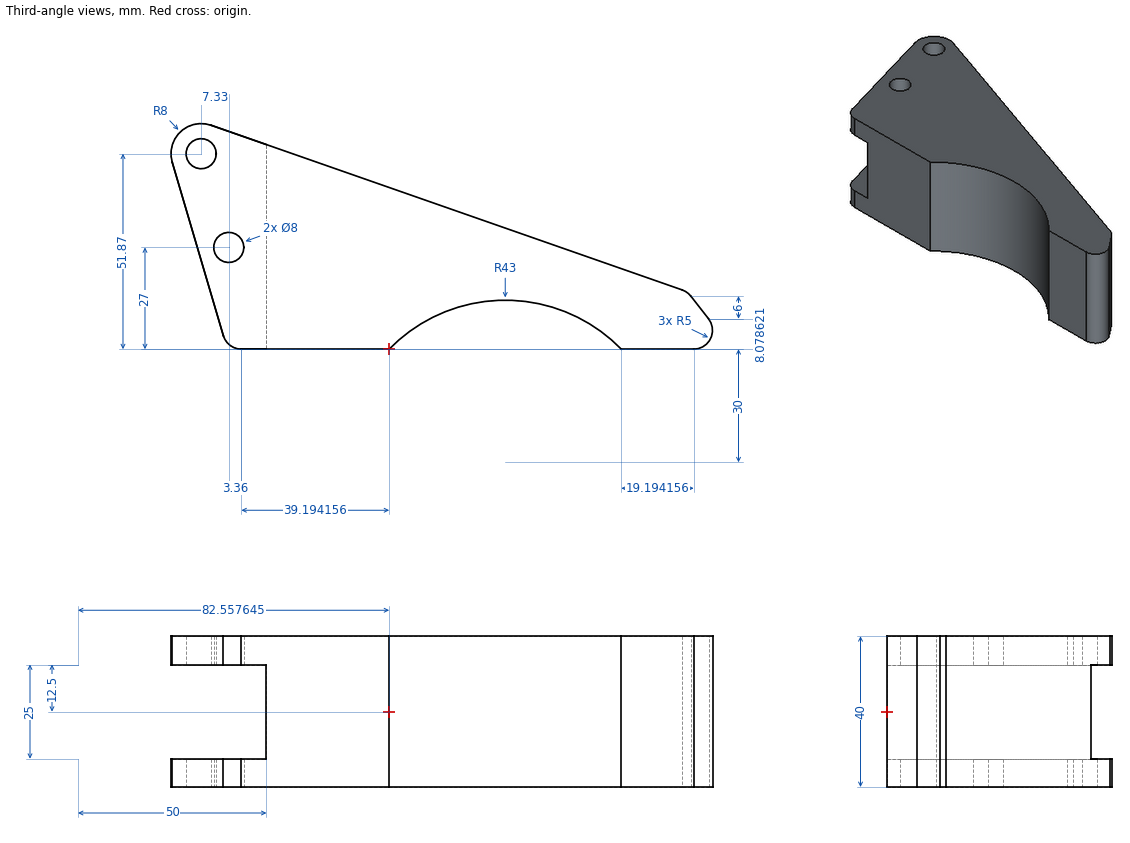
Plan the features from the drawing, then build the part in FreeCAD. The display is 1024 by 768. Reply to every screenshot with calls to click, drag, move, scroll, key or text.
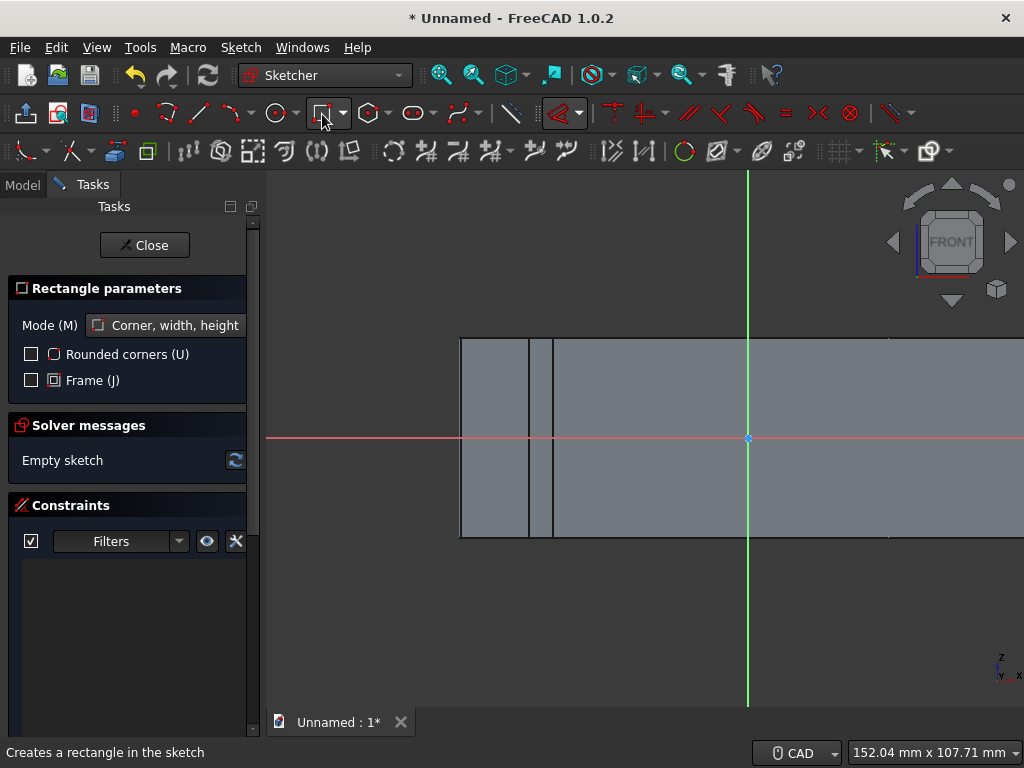
click(336, 376)
click(586, 500)
key(Escape)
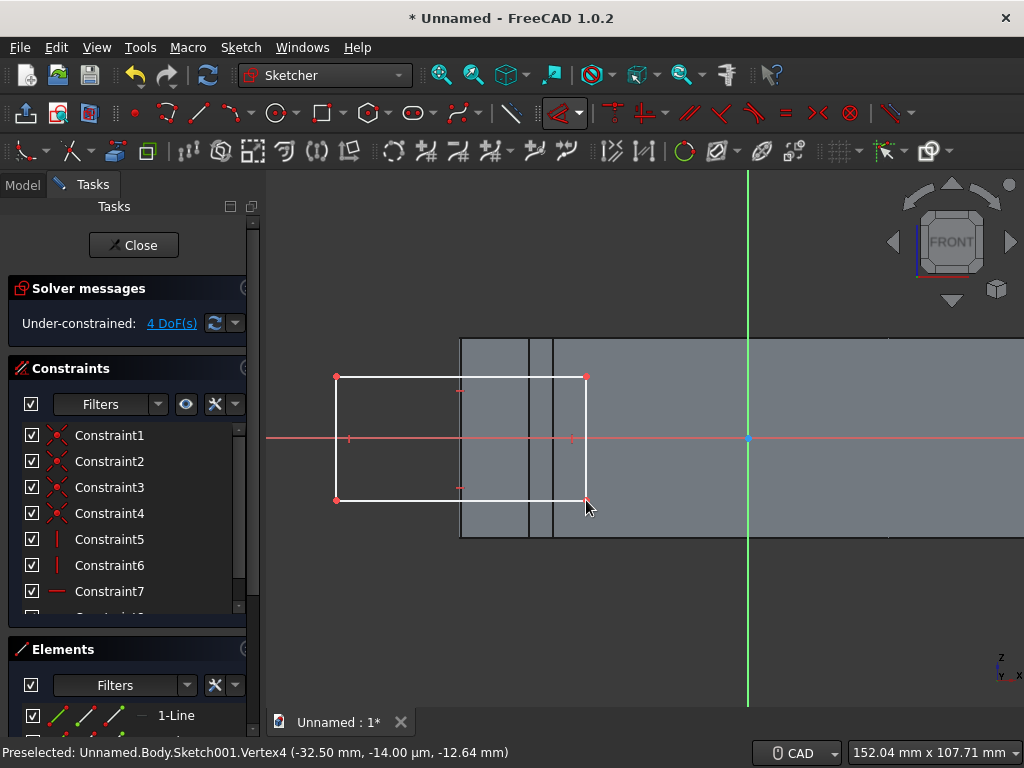
click(336, 414)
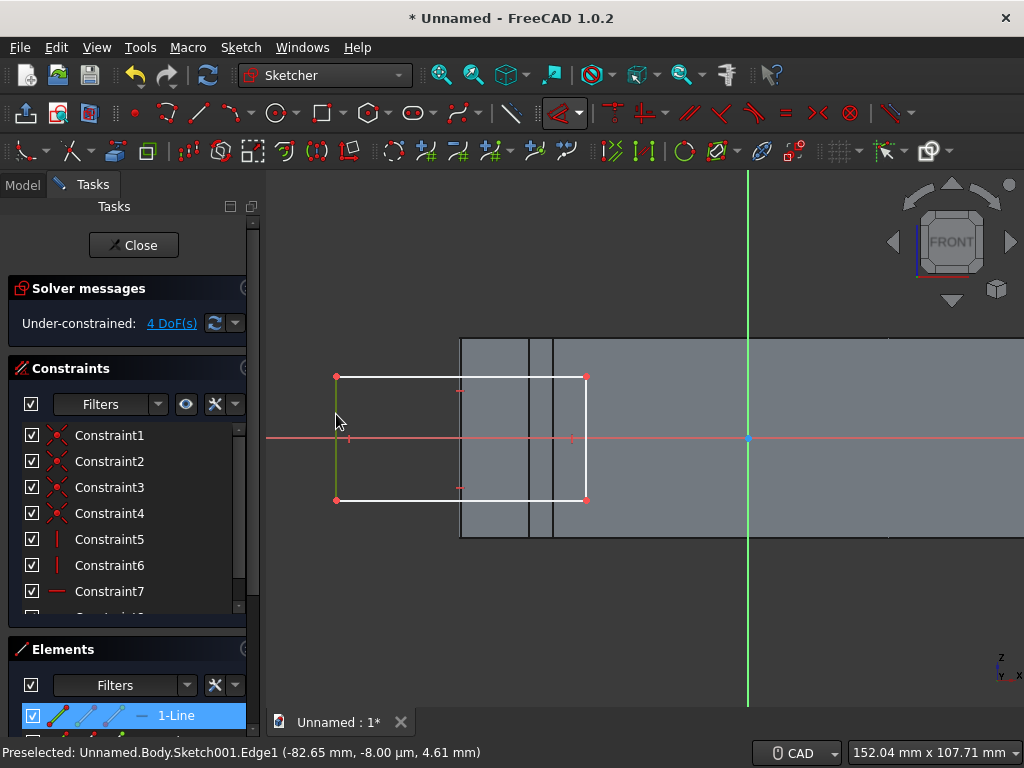
key(i)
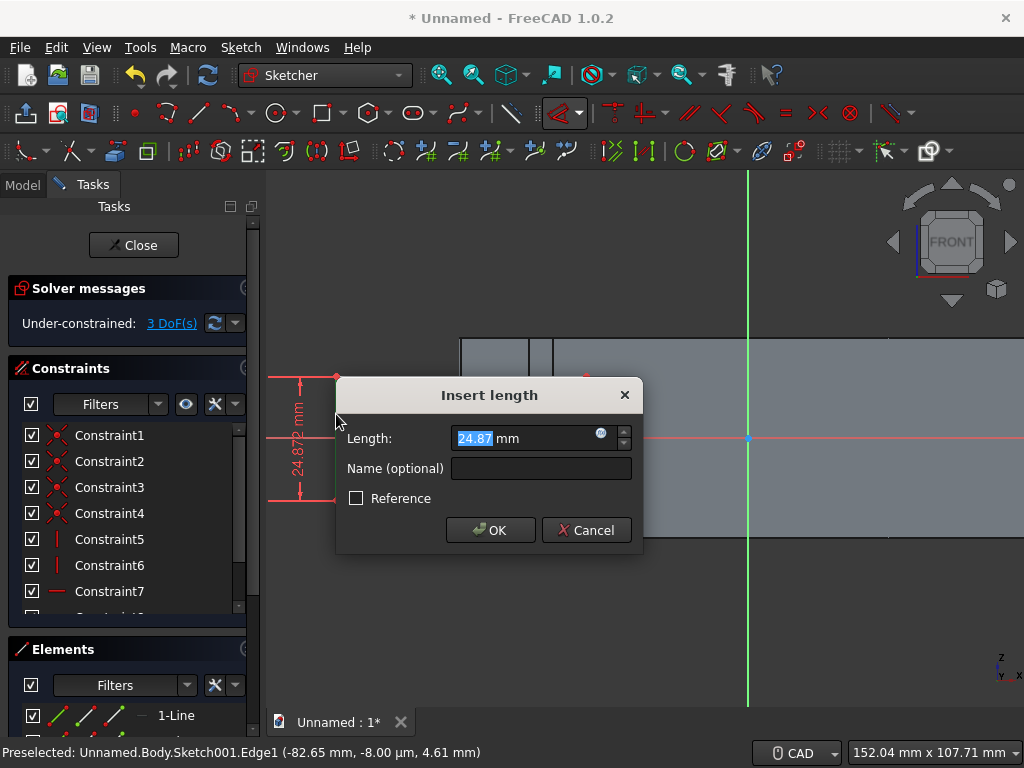
text(25)
key(Return)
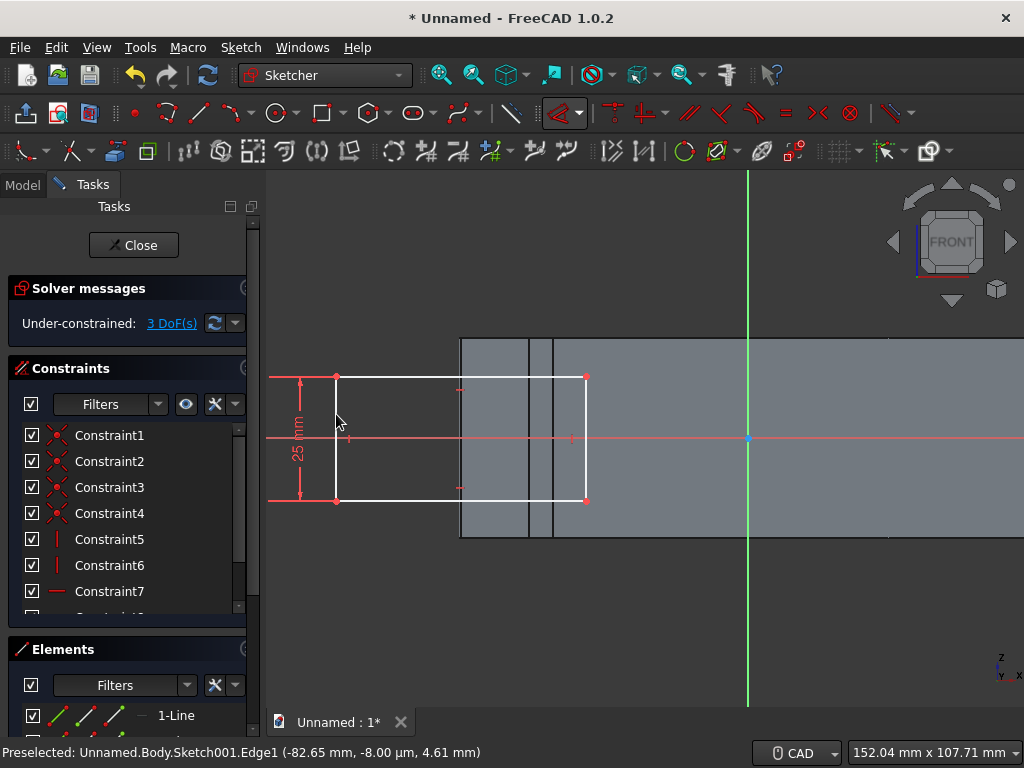
click(411, 501)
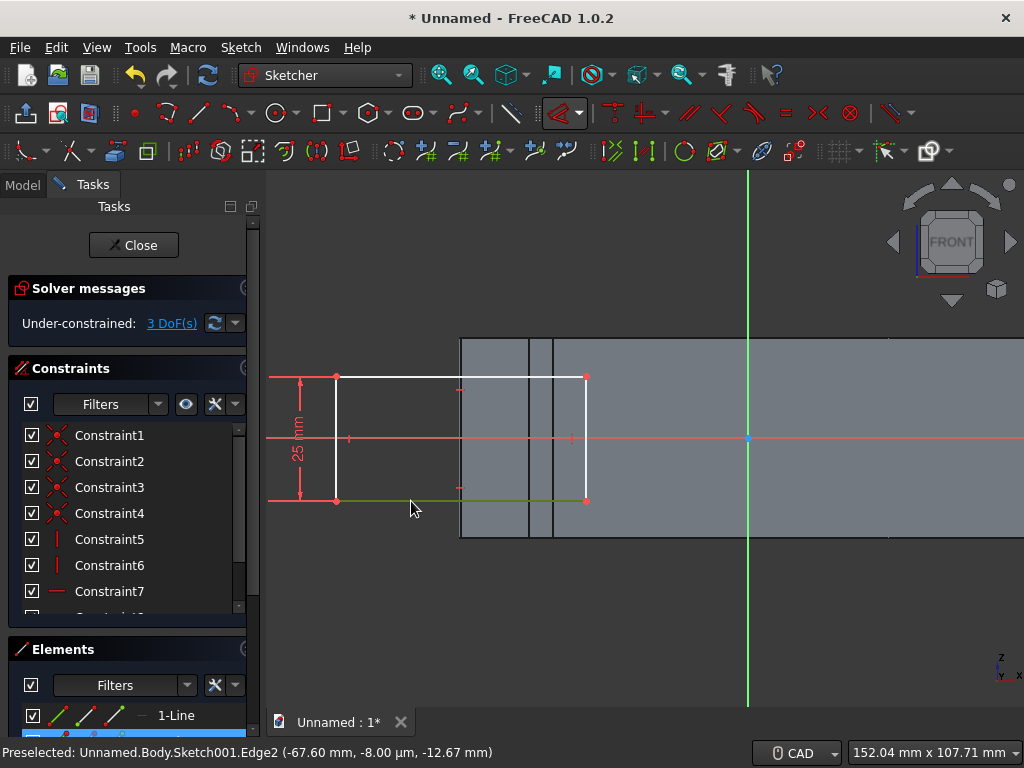
key(l)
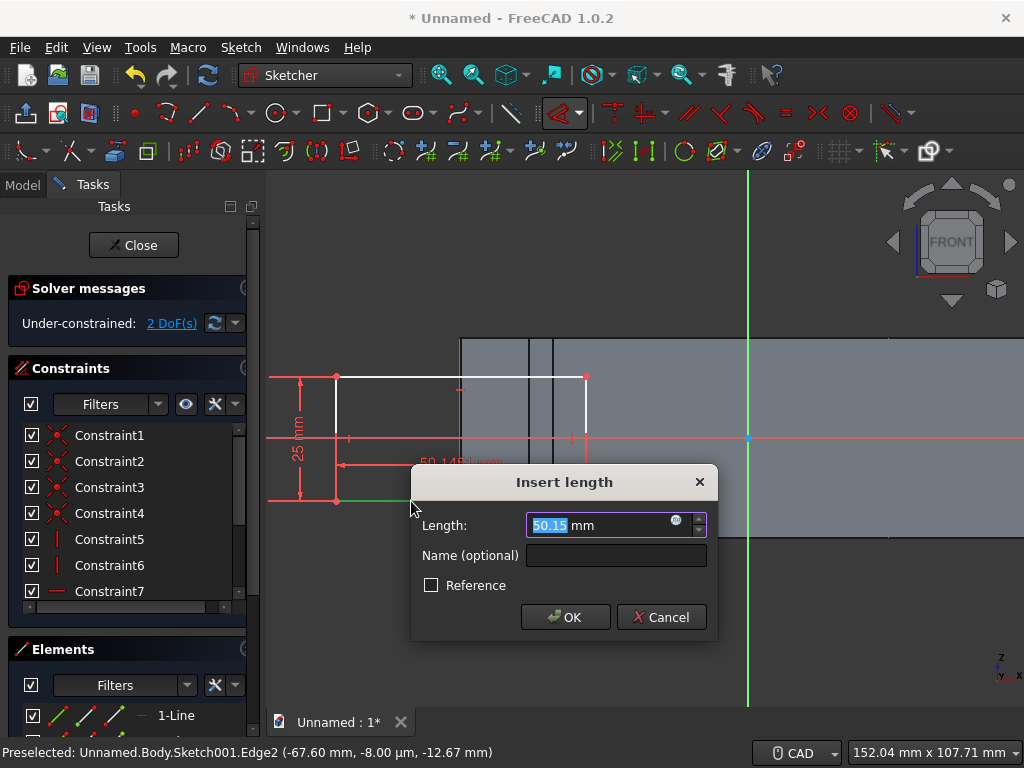
text(50)
key(Return)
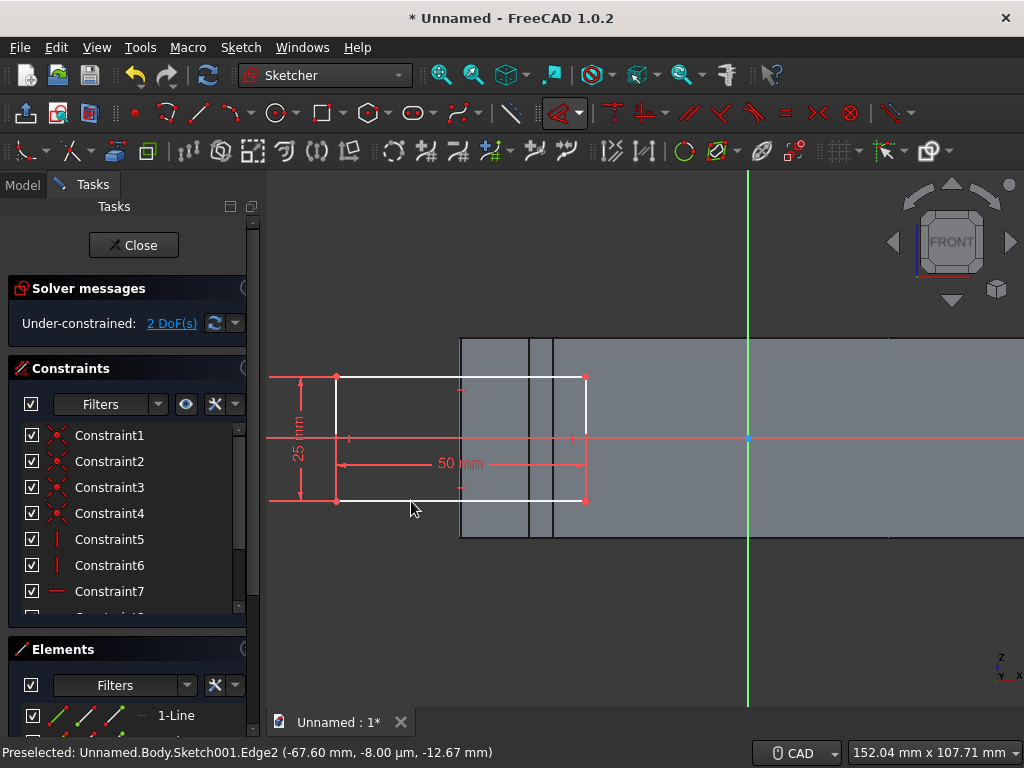
click(336, 377)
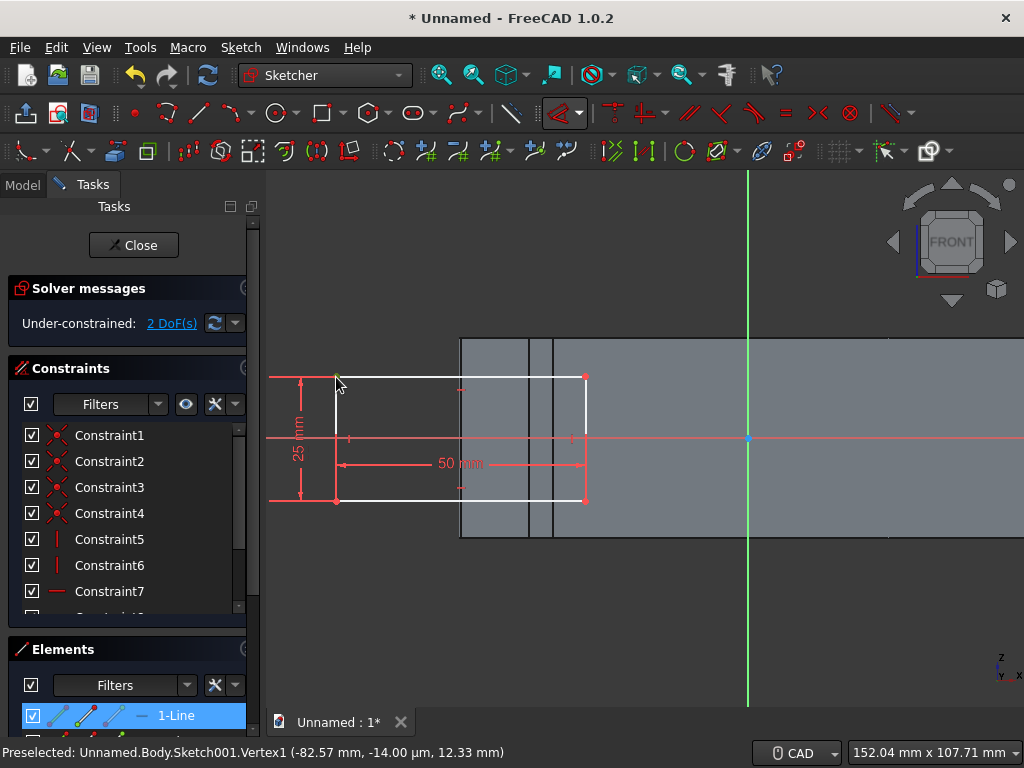
key(i)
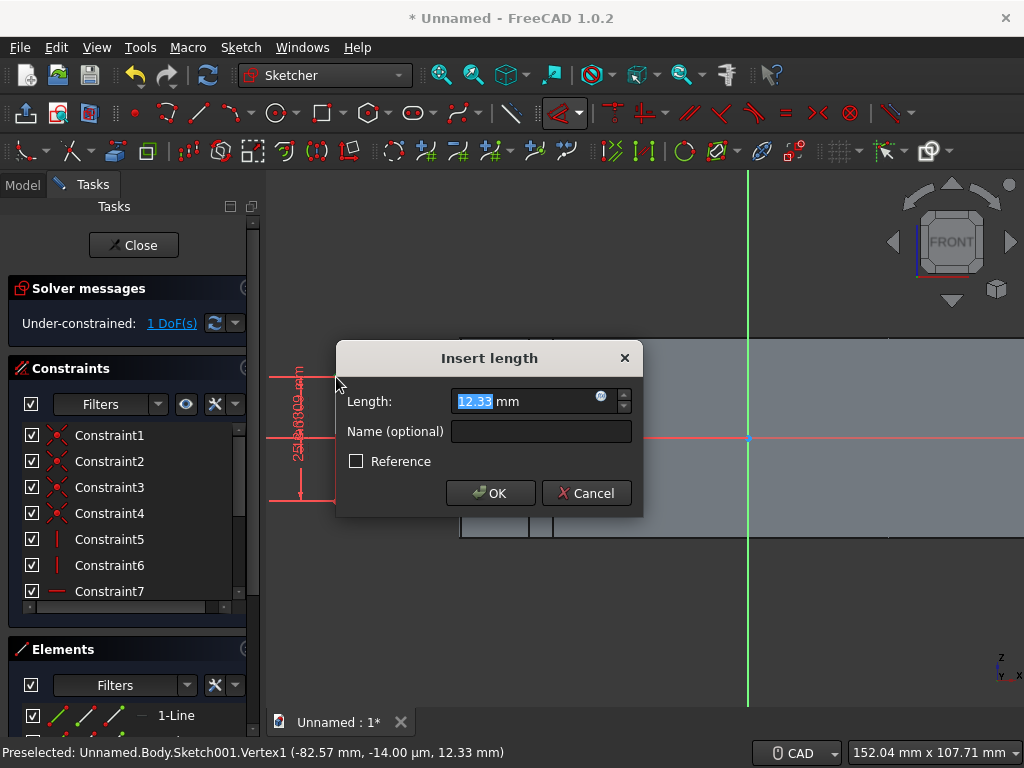
text(12.5)
key(Return)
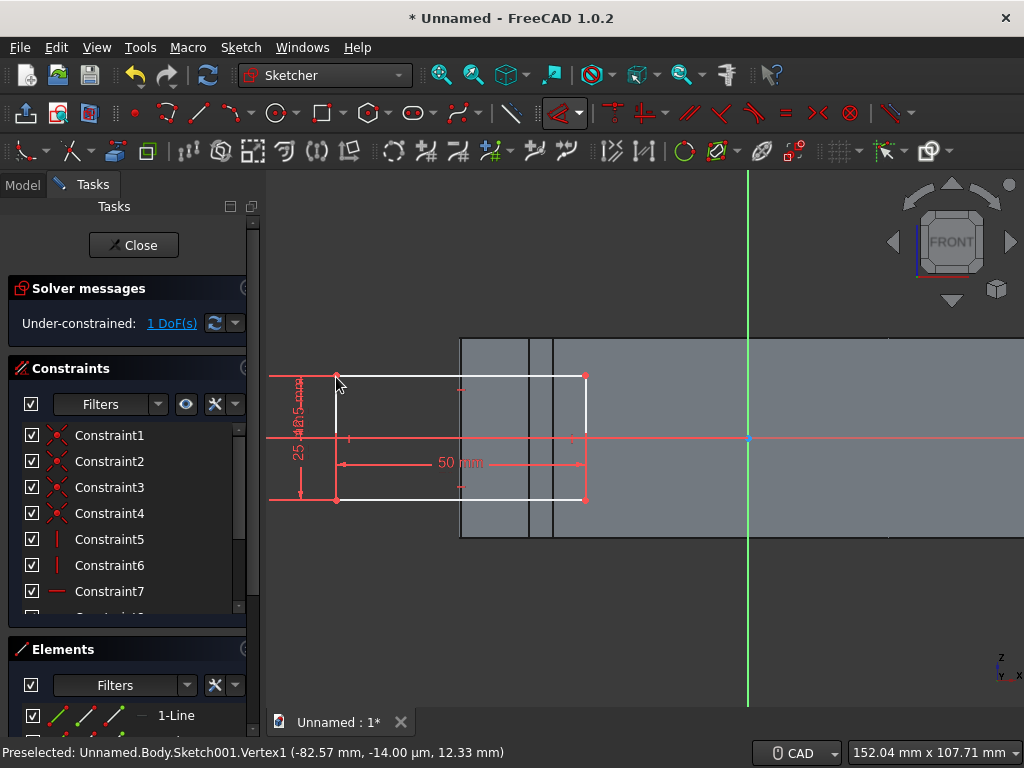
click(336, 376)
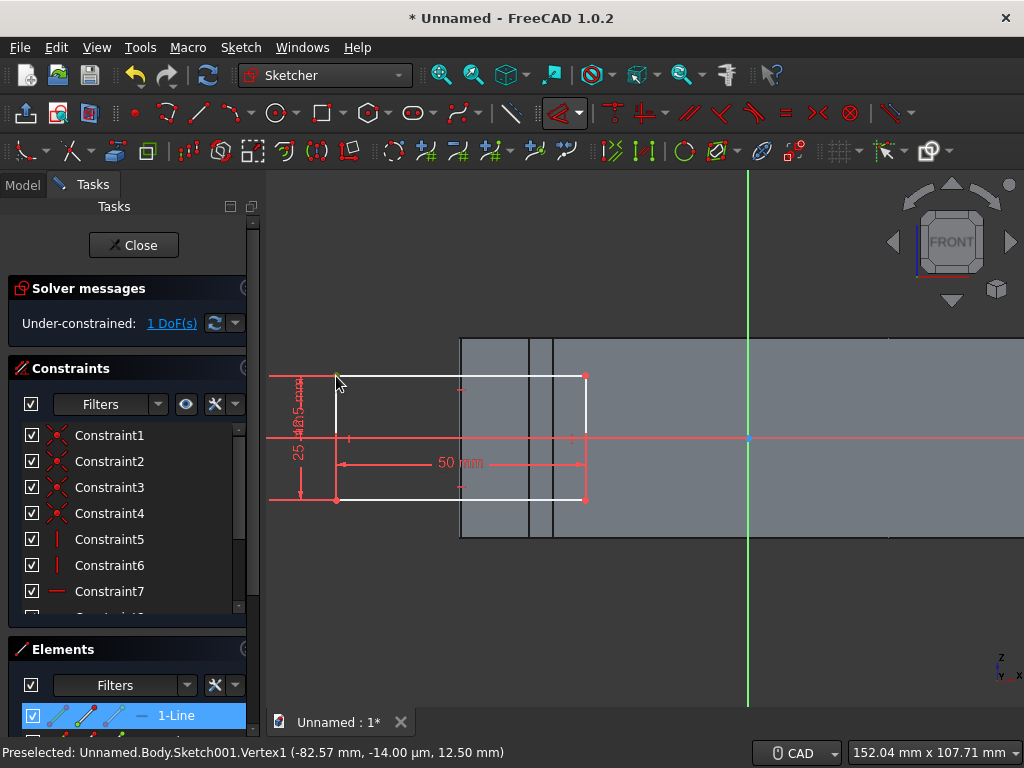
key(l)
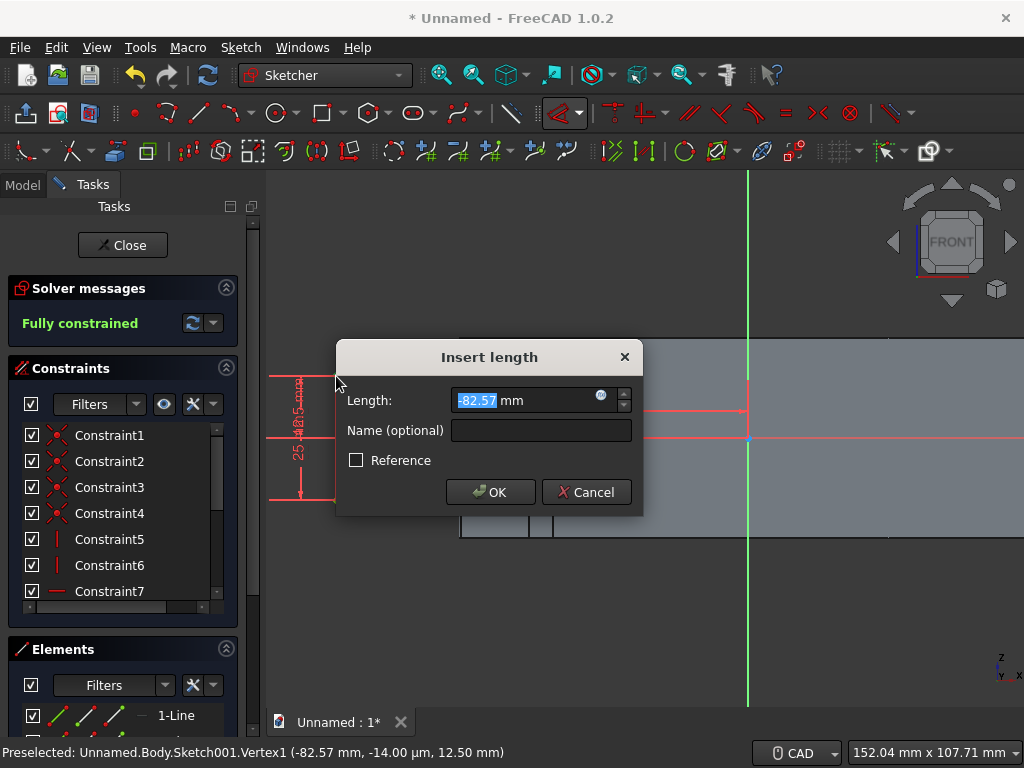
text(-82.557645)
key(Return)